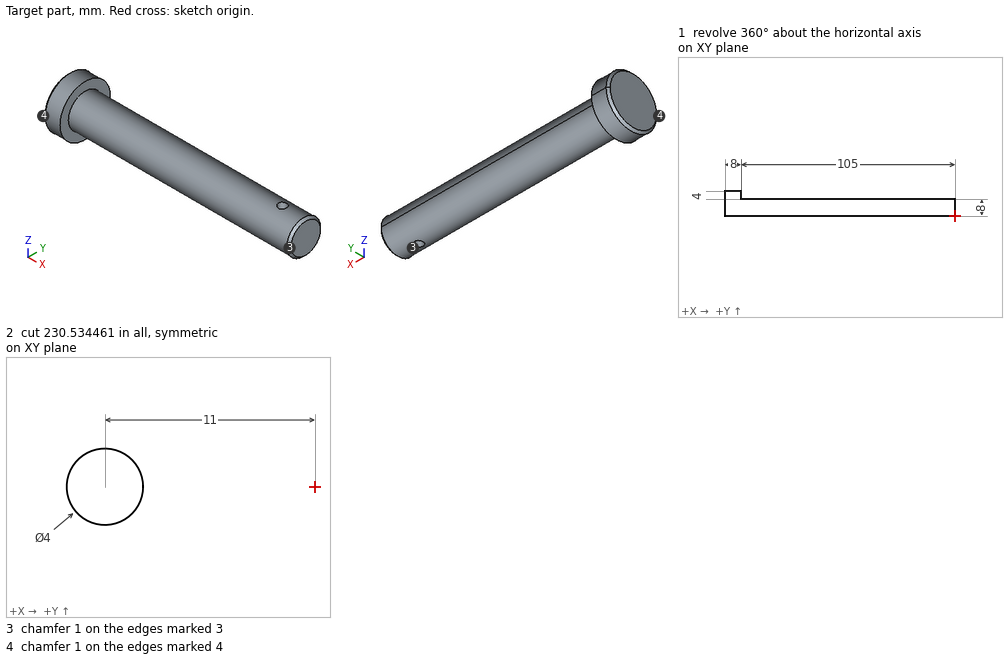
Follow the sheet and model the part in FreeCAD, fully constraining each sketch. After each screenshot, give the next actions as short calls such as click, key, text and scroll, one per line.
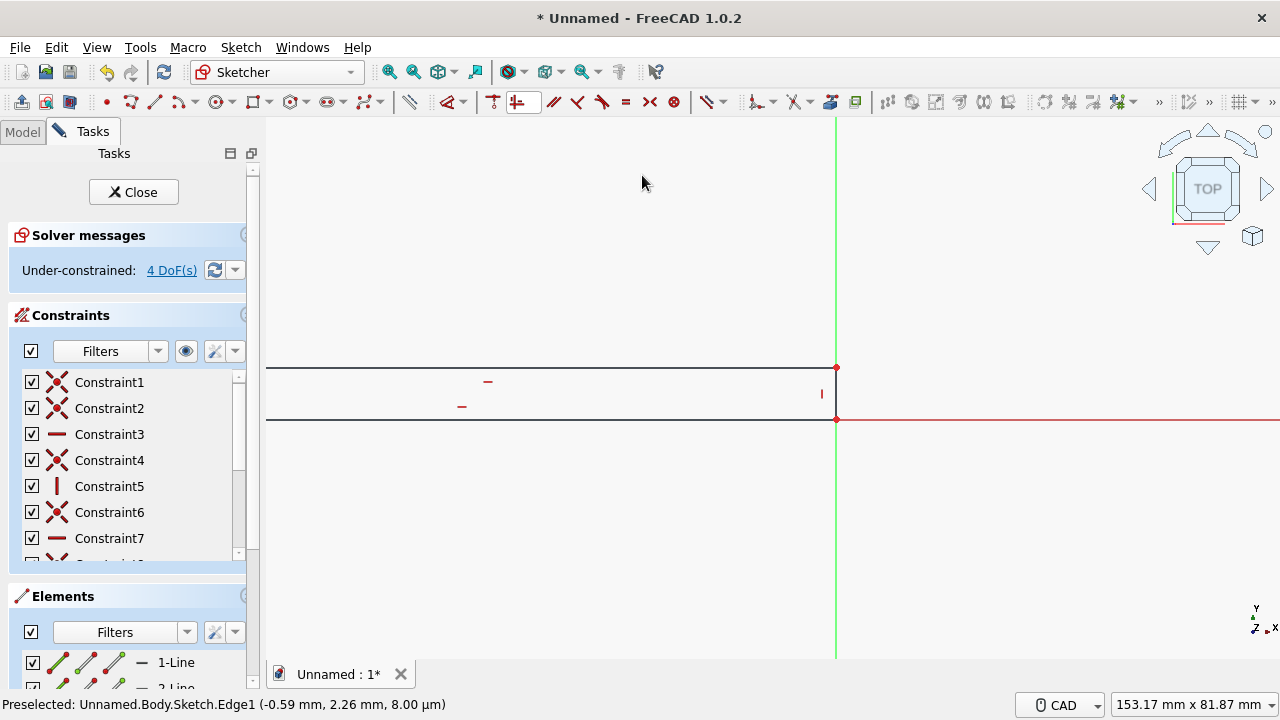
click(836, 404)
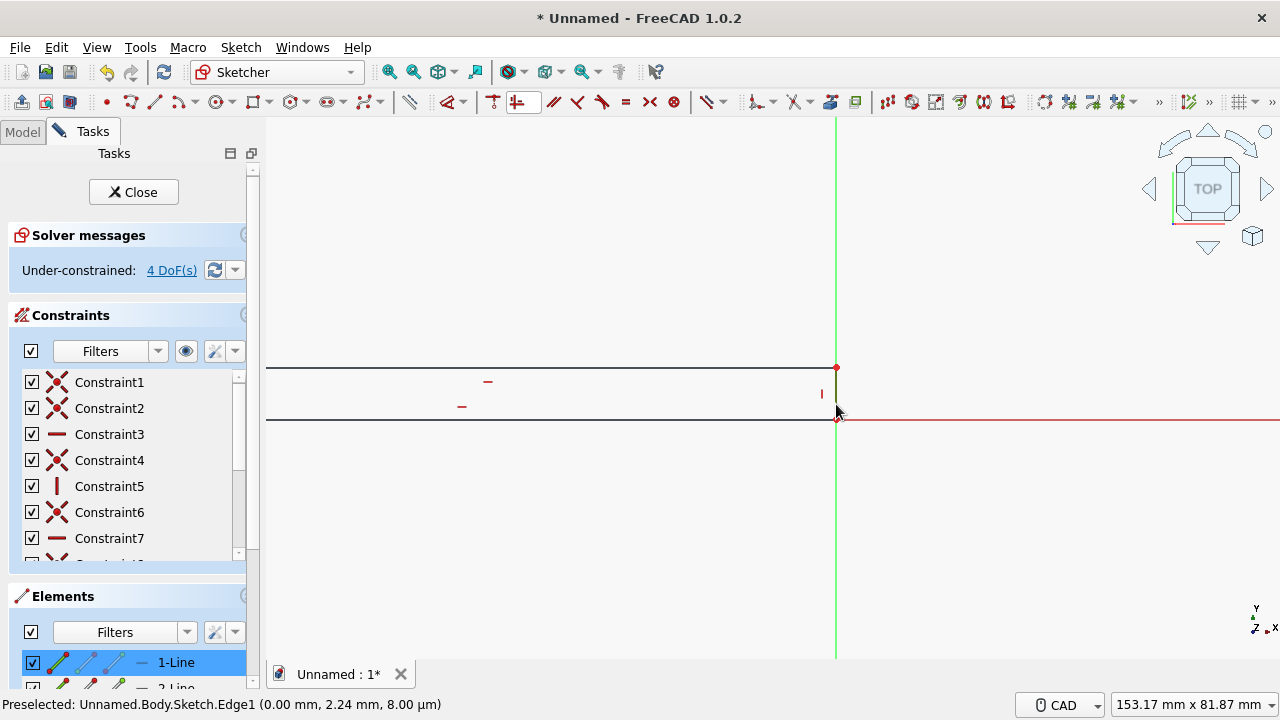
key(i)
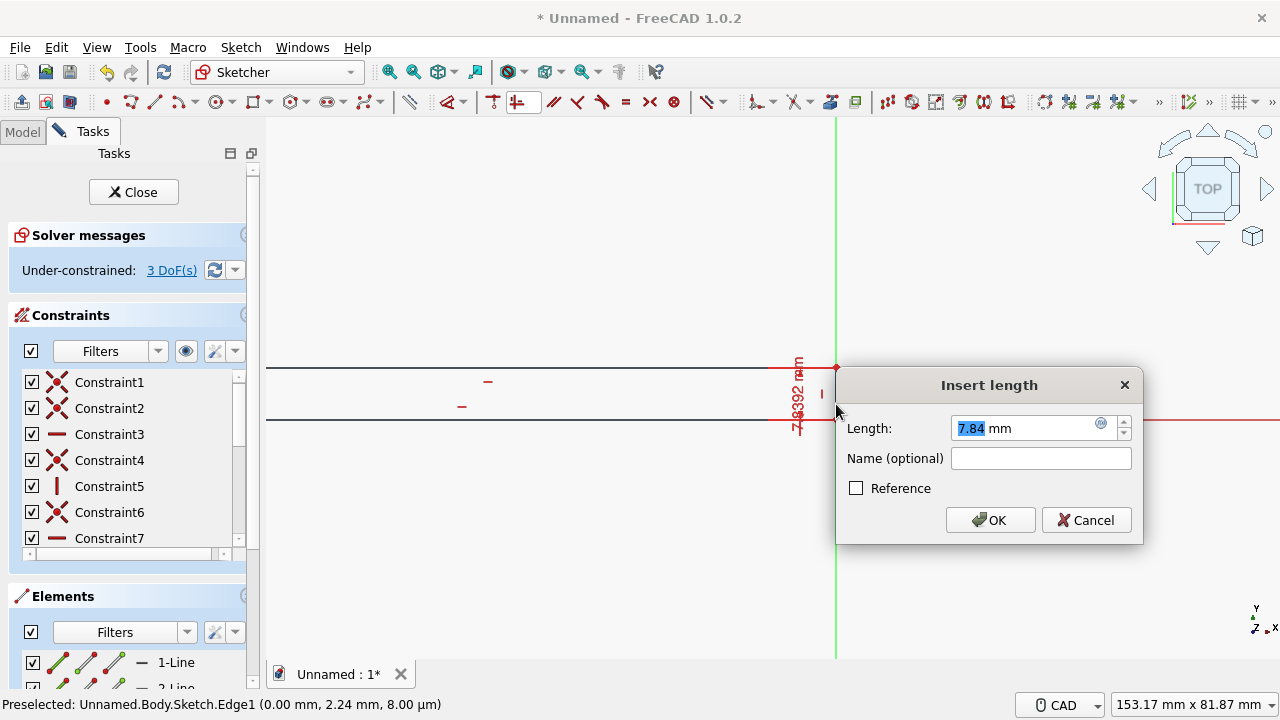
text(8)
key(Return)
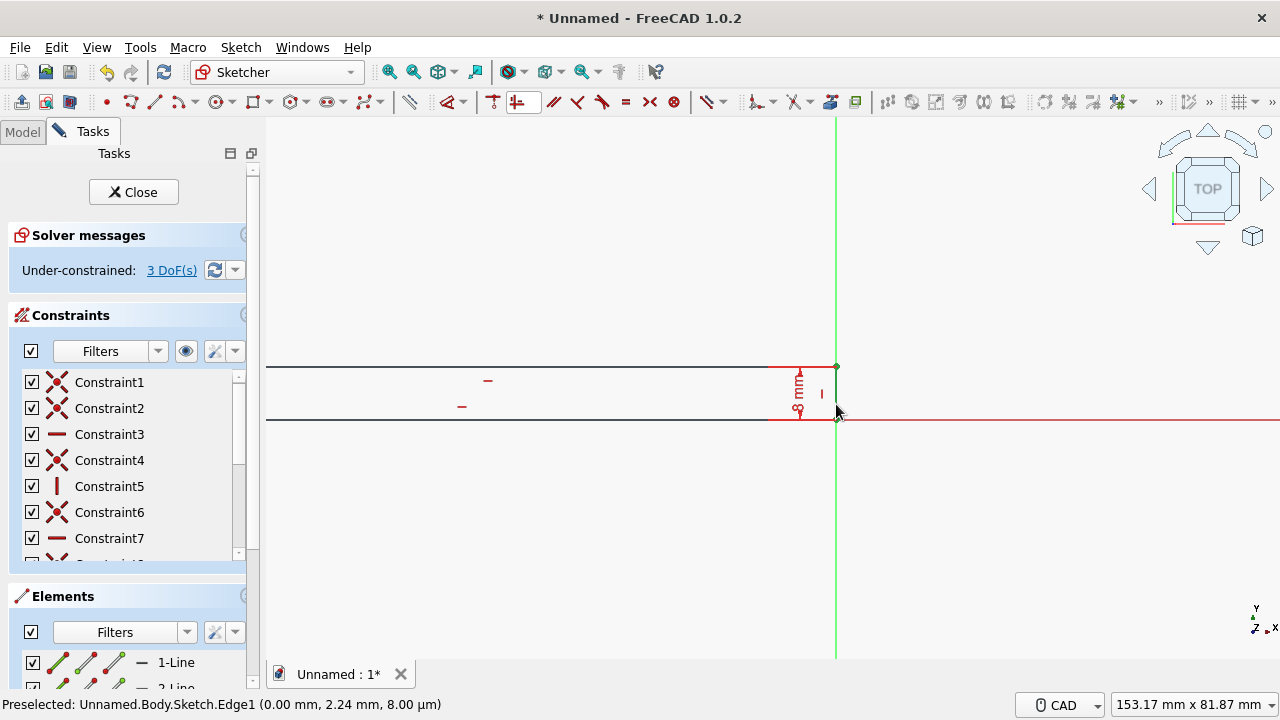
scroll(1115, 404, down, 2)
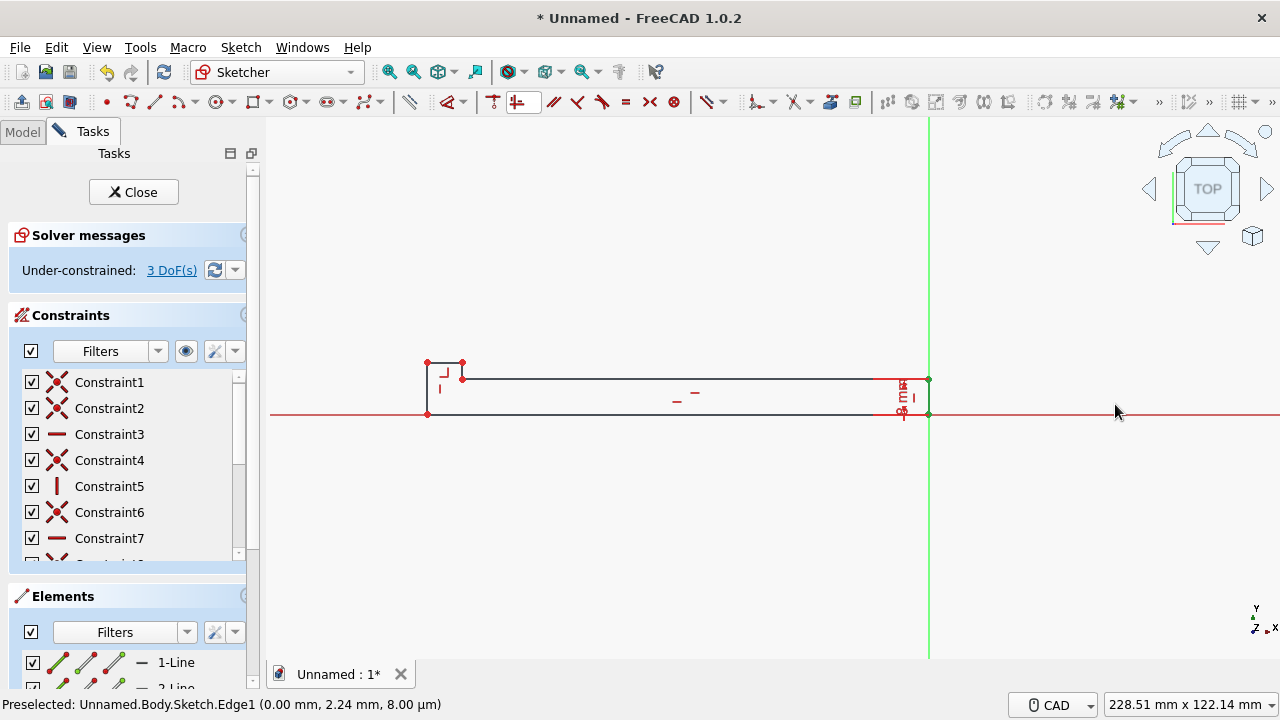
scroll(462, 373, up, 5)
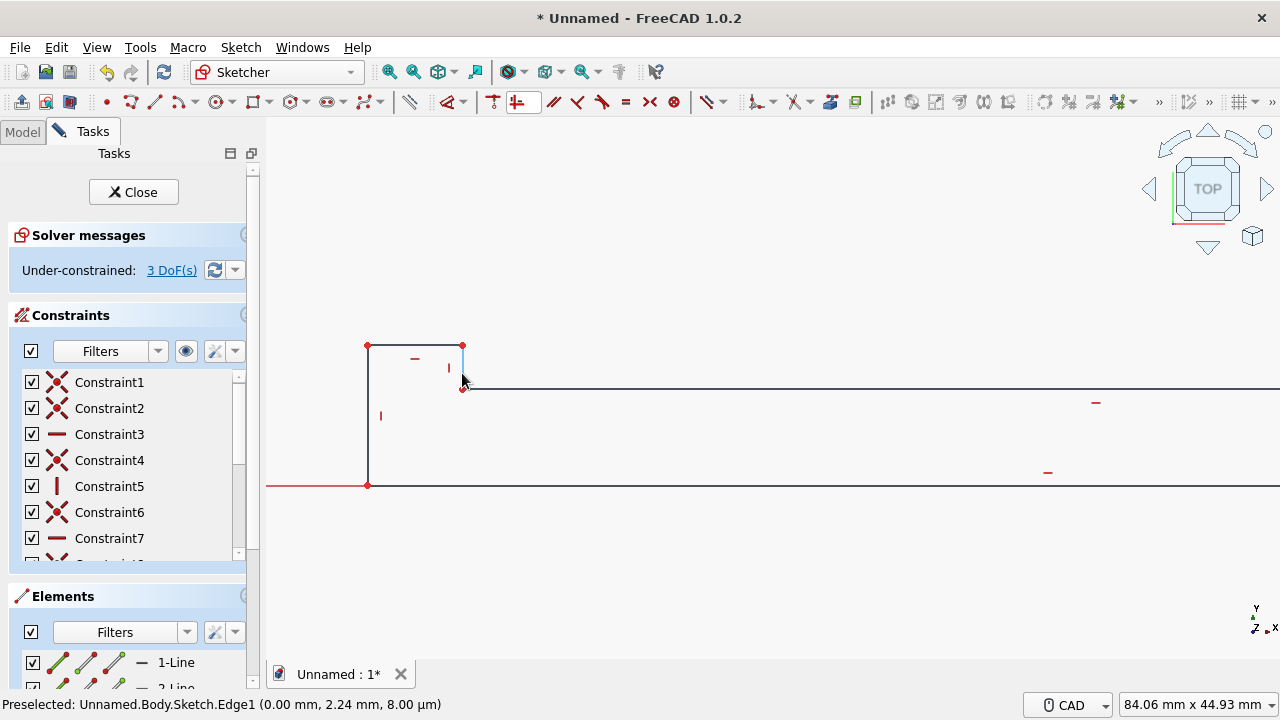
click(463, 372)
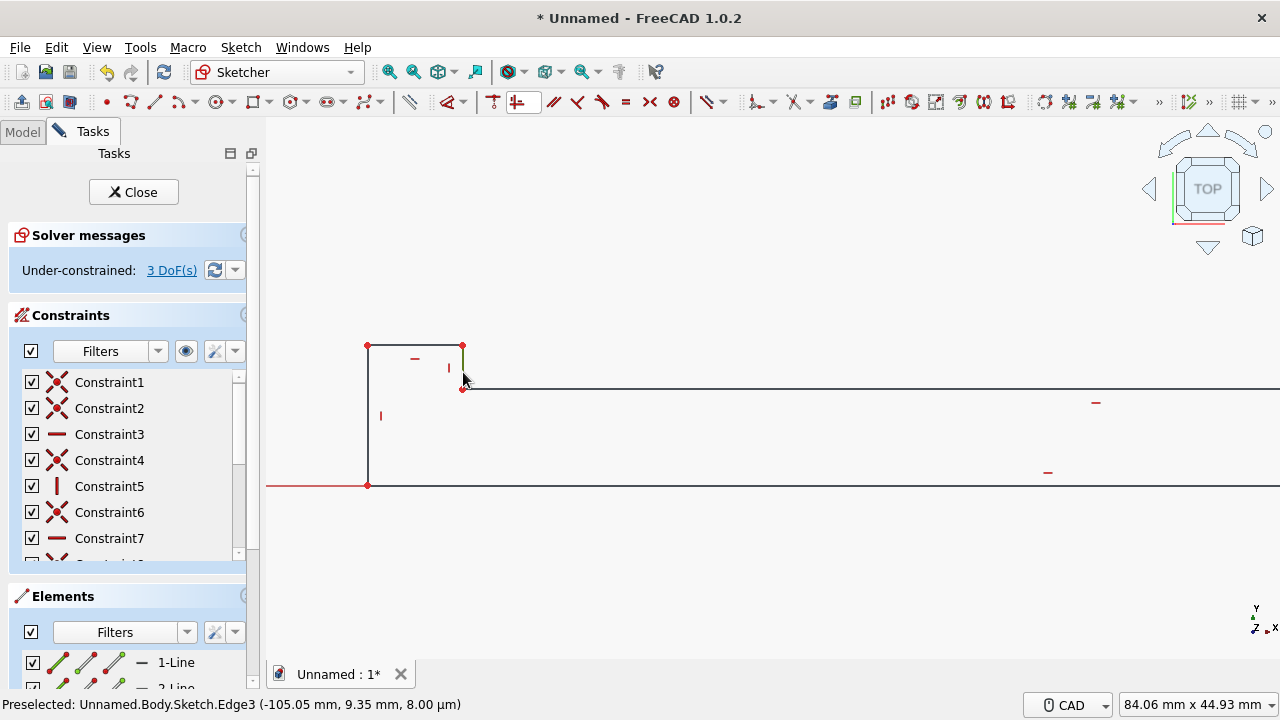
key(i)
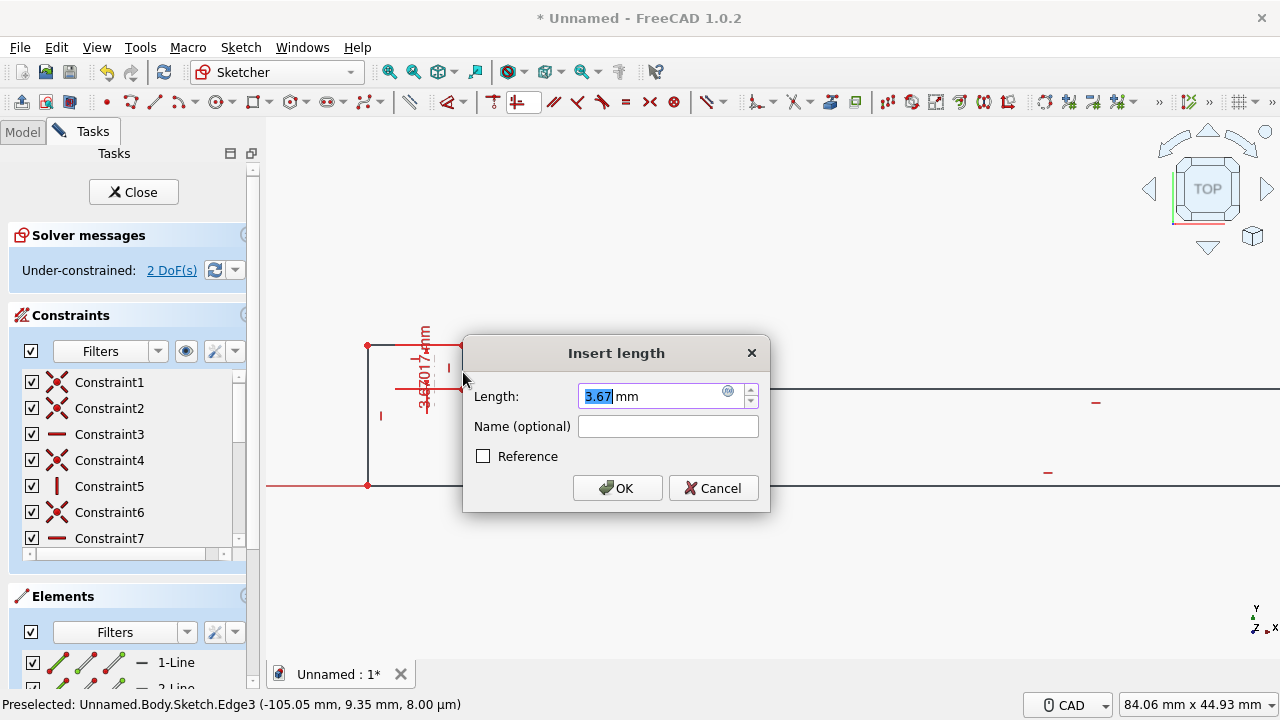
text(4)
key(Return)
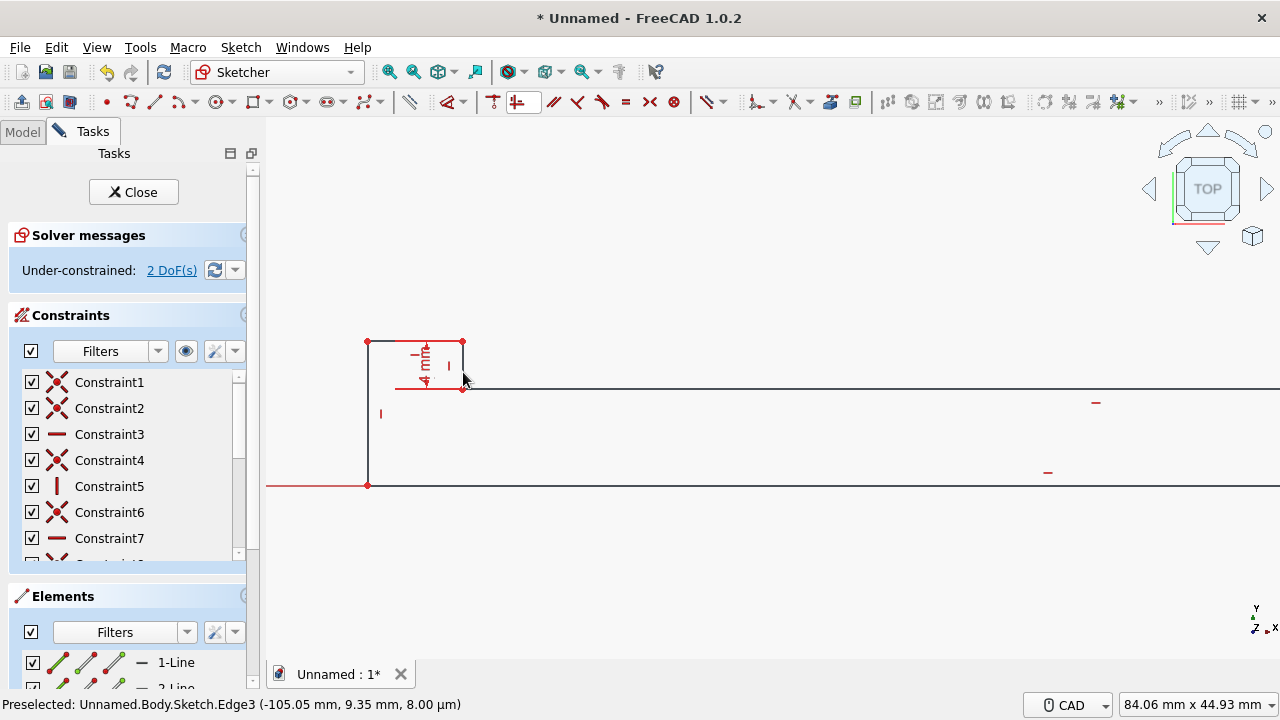
click(434, 341)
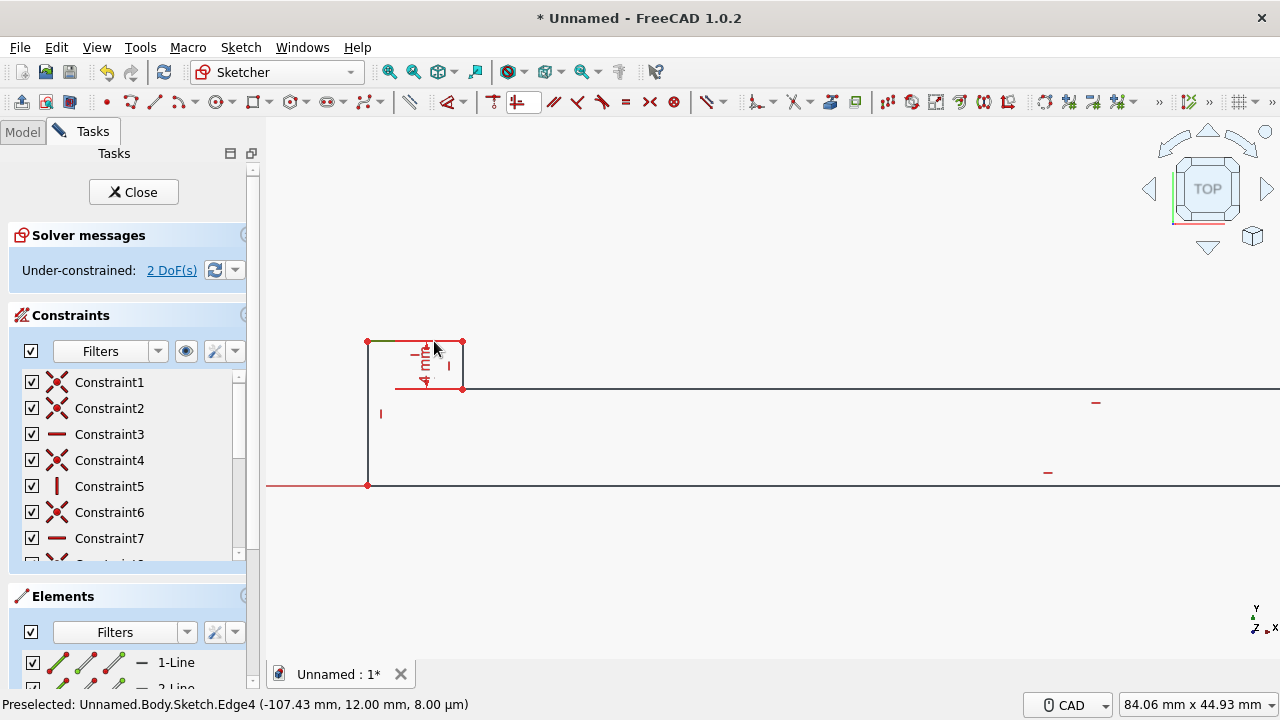
click(466, 102)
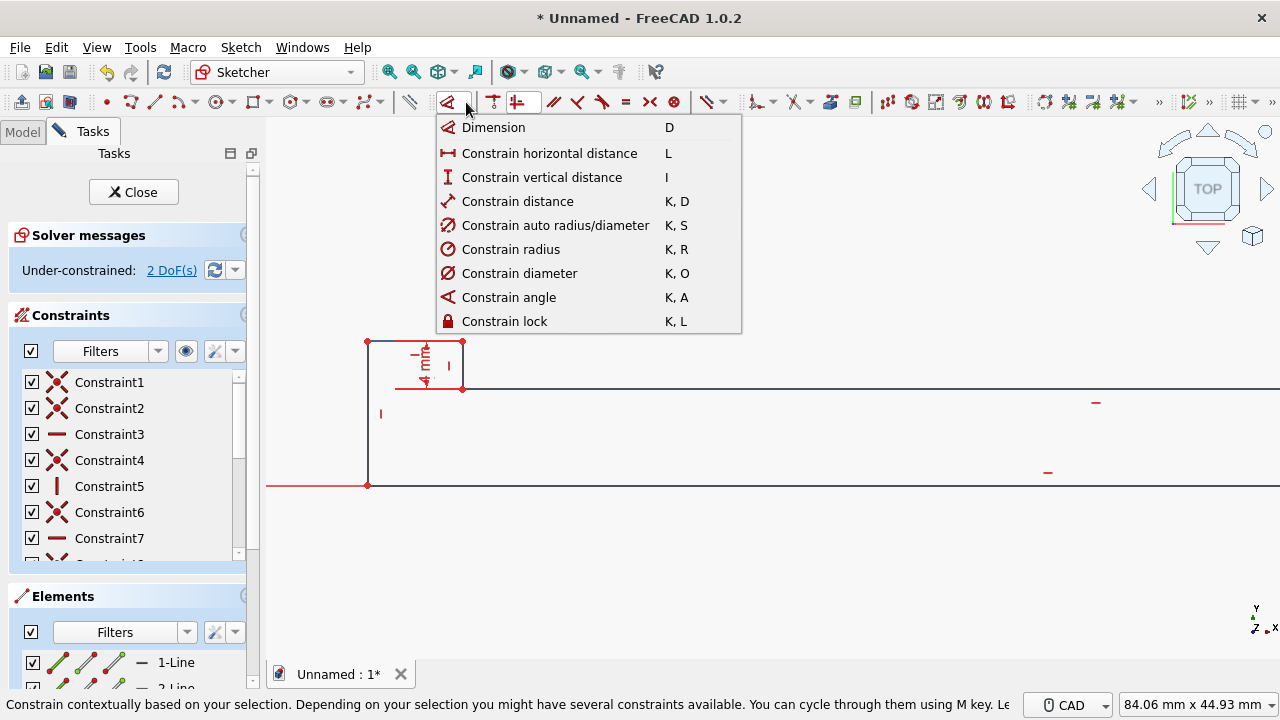
click(589, 153)